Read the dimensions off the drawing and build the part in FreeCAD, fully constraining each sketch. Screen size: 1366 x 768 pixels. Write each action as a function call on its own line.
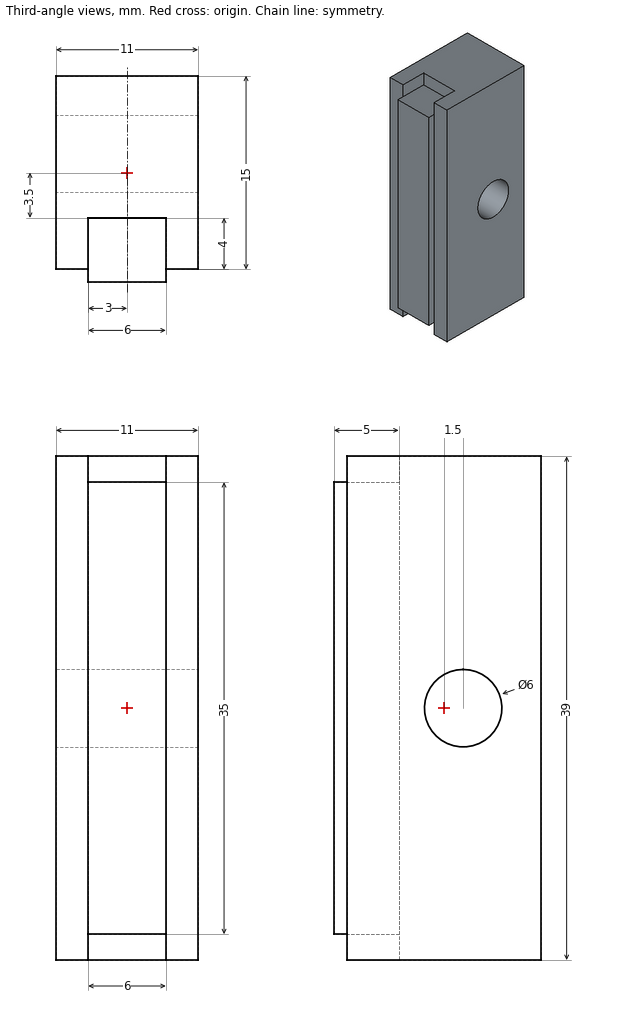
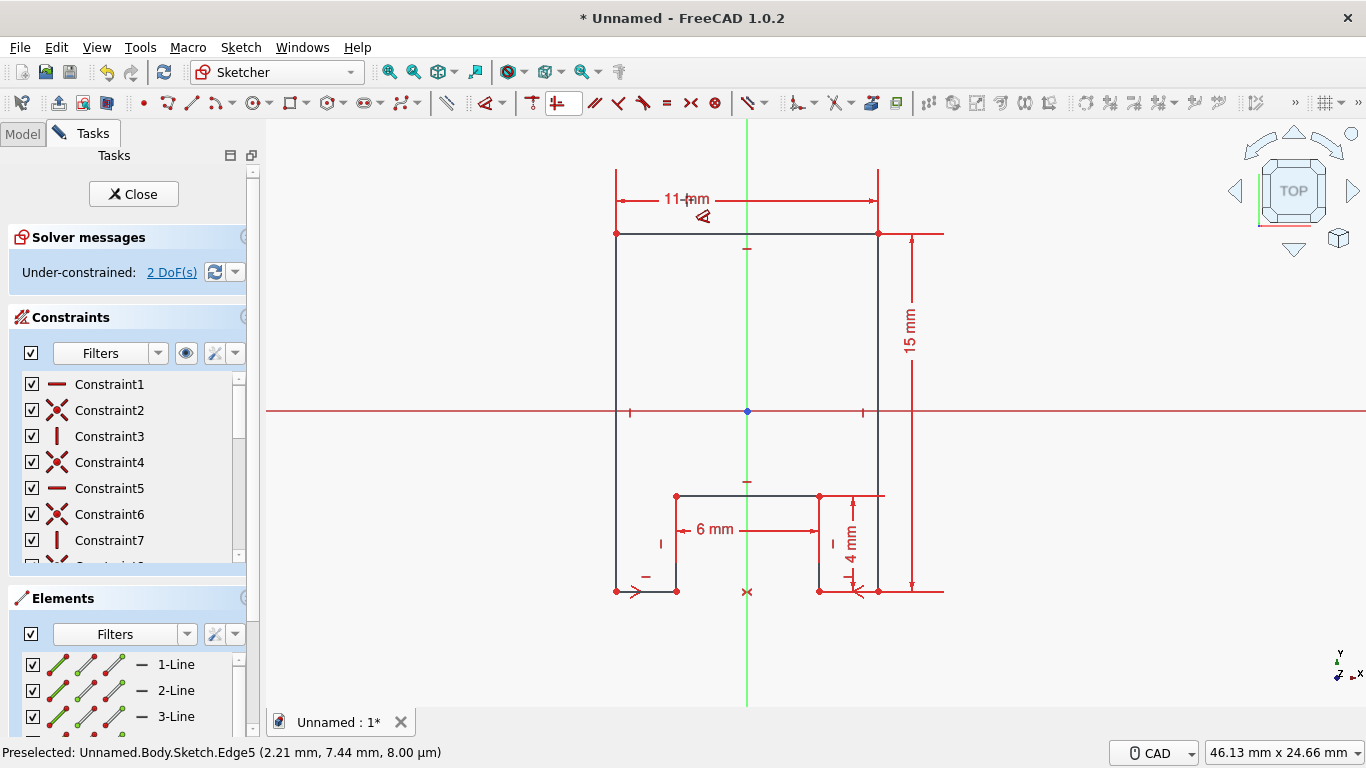
click(676, 496)
click(712, 377)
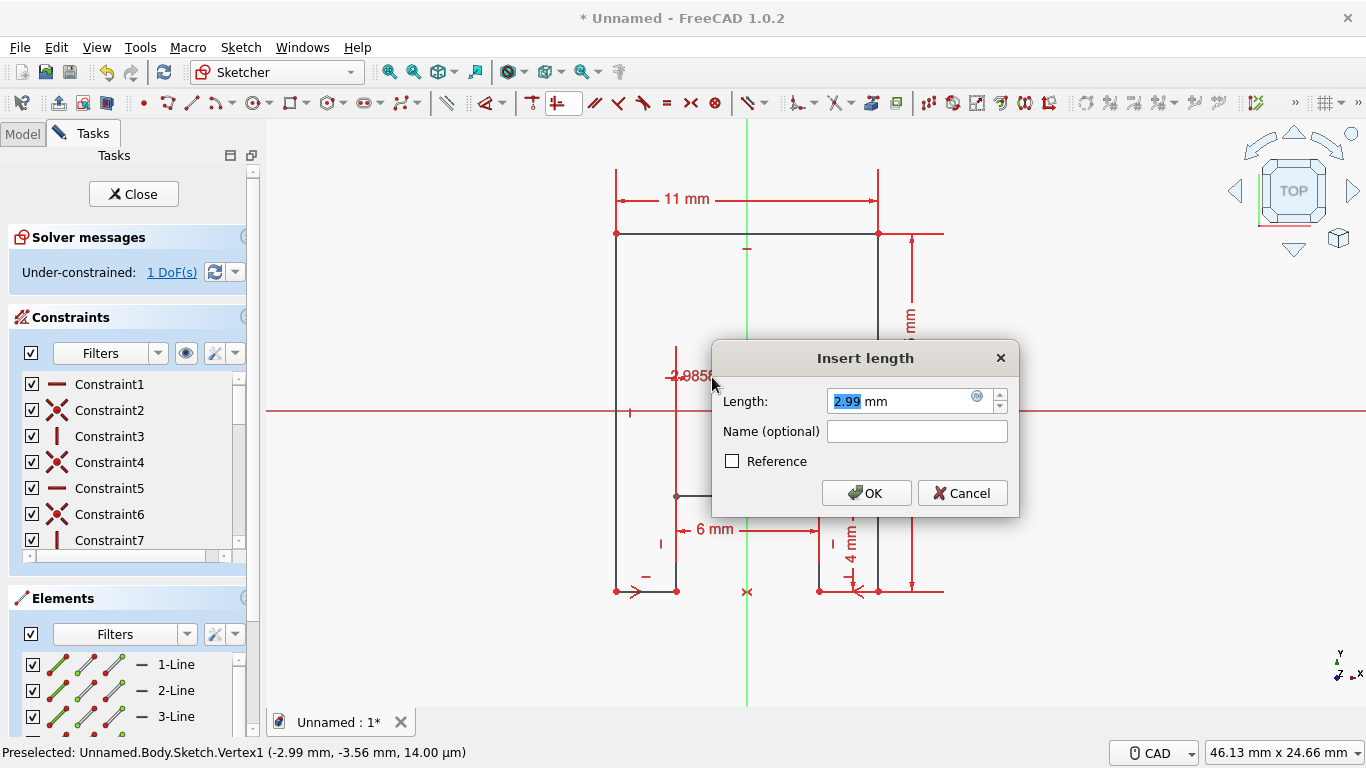
text(3)
key(Return)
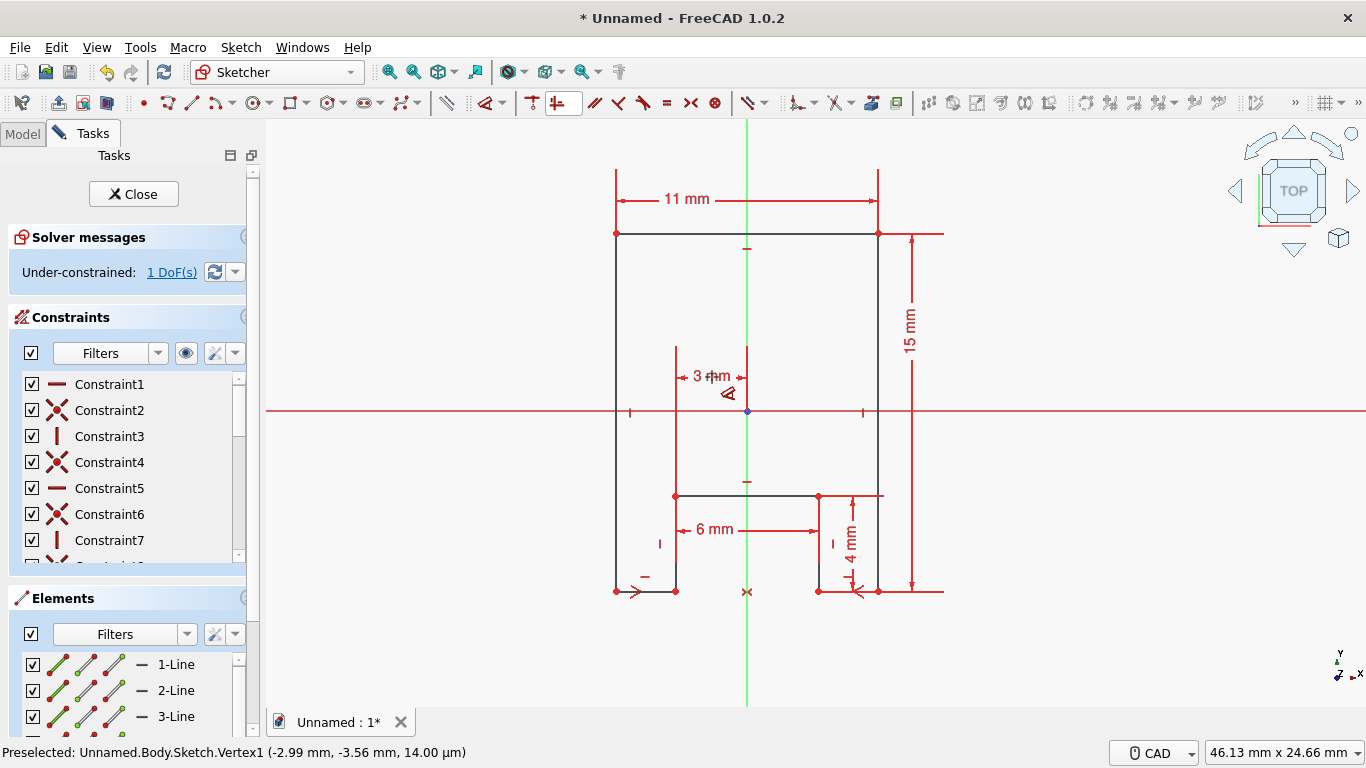
click(676, 496)
click(642, 454)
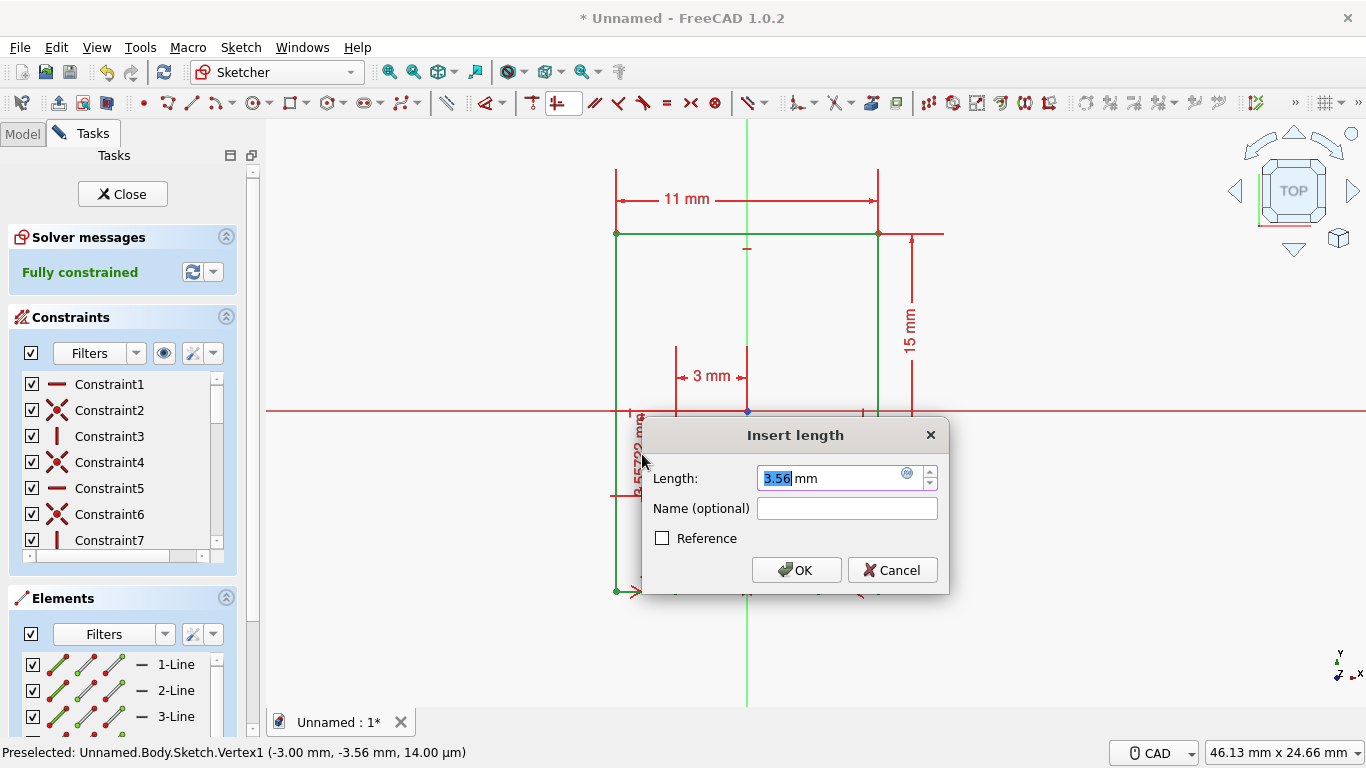
text(3.5)
key(Return)
key(Escape)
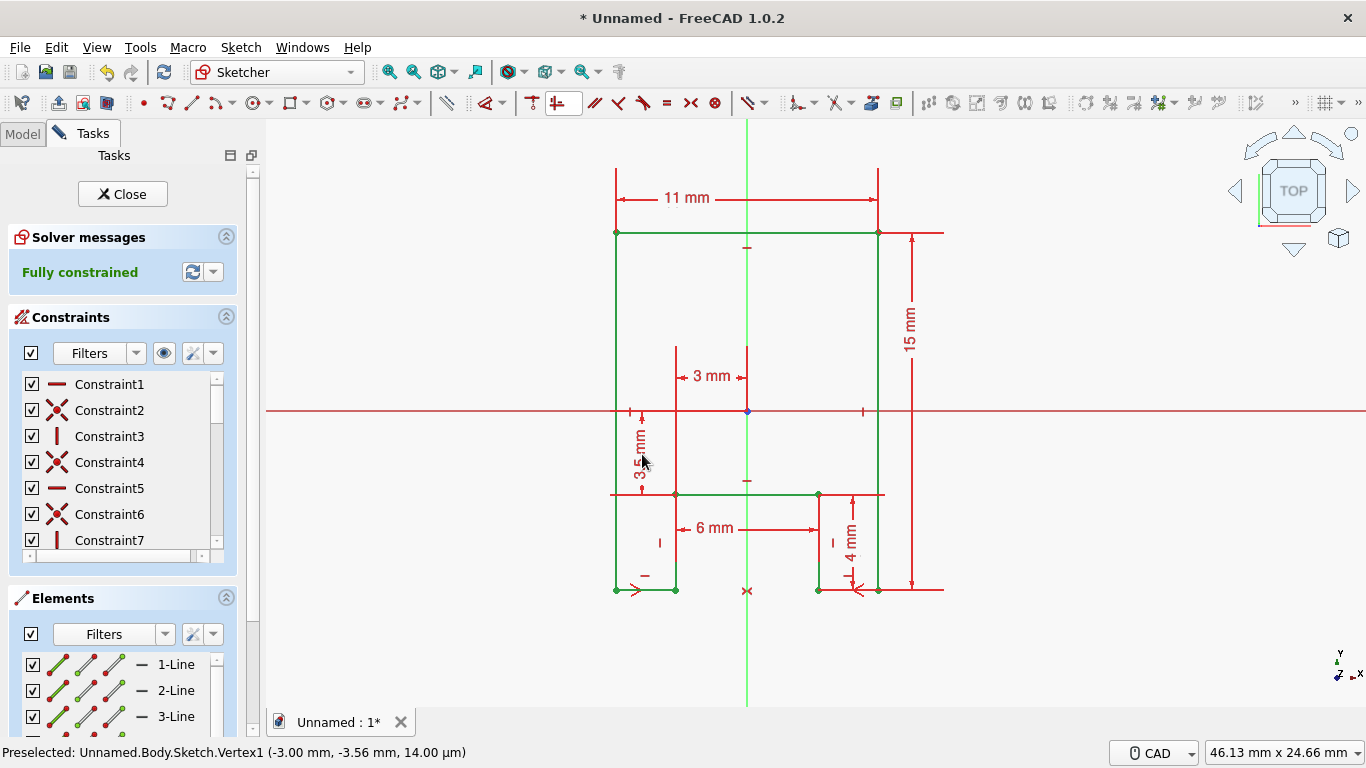
click(123, 194)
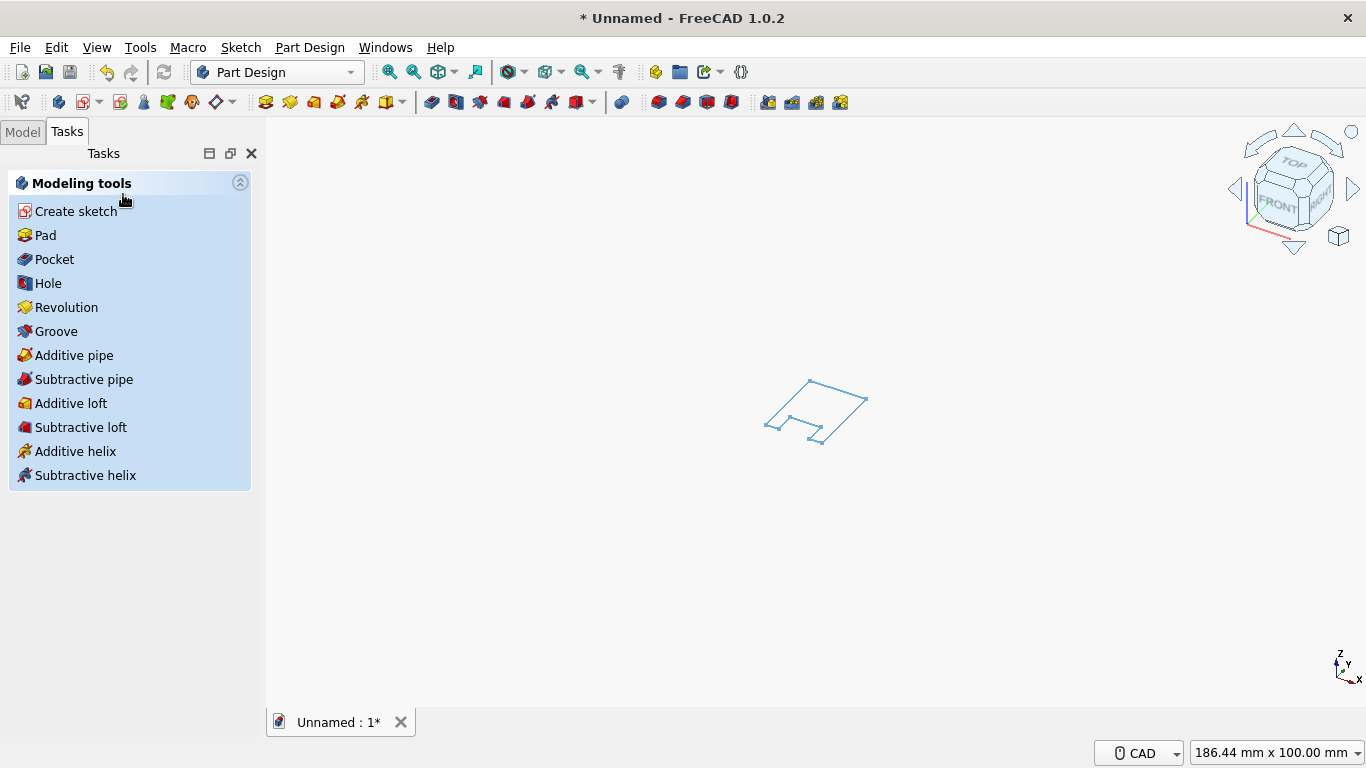
click(266, 102)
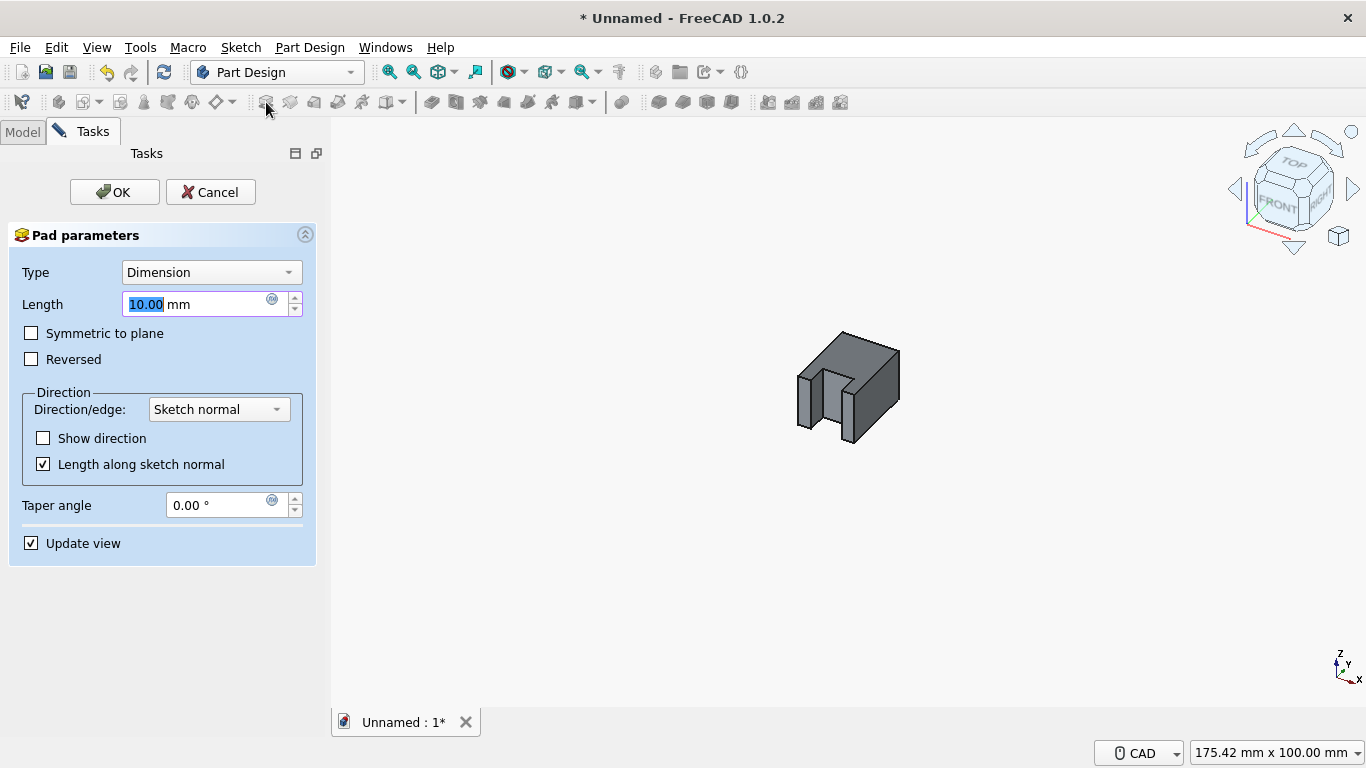
text(39)
key(Tab)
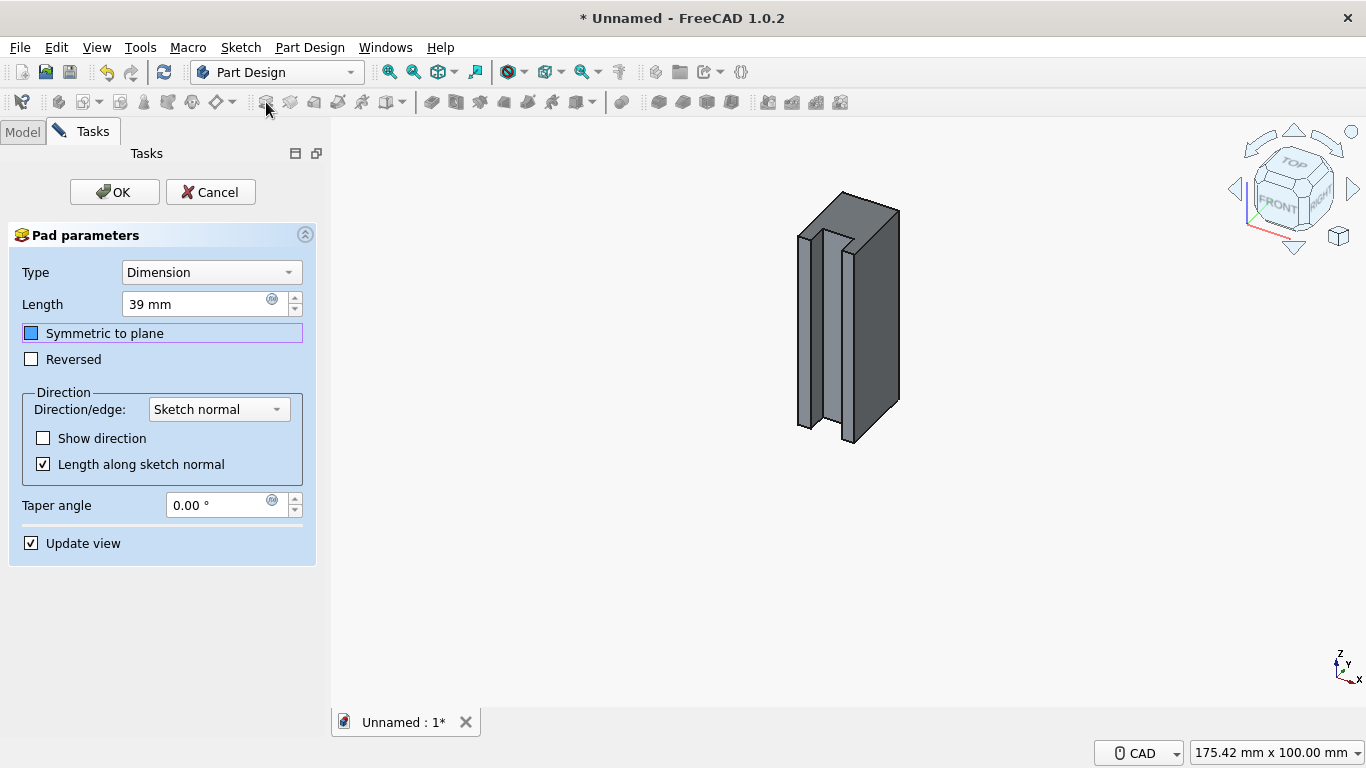
click(30, 333)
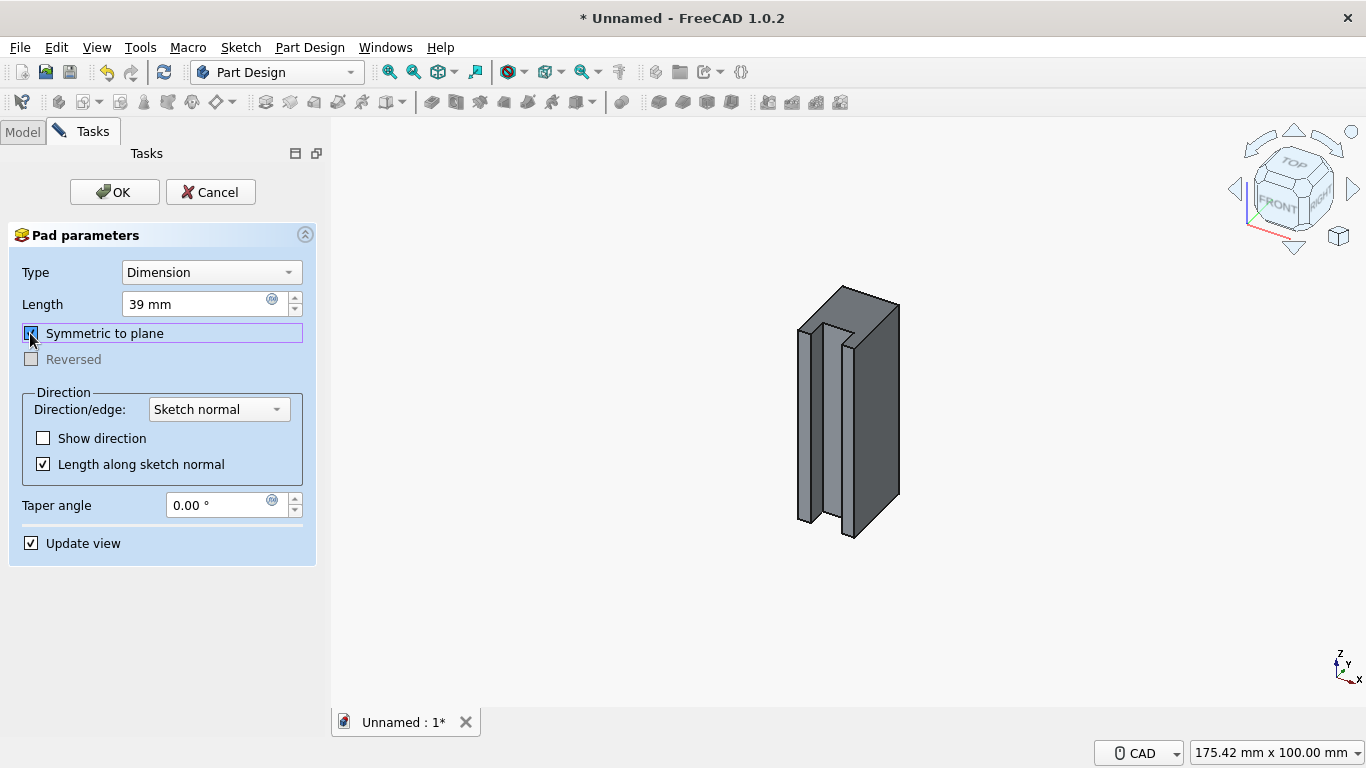
click(115, 192)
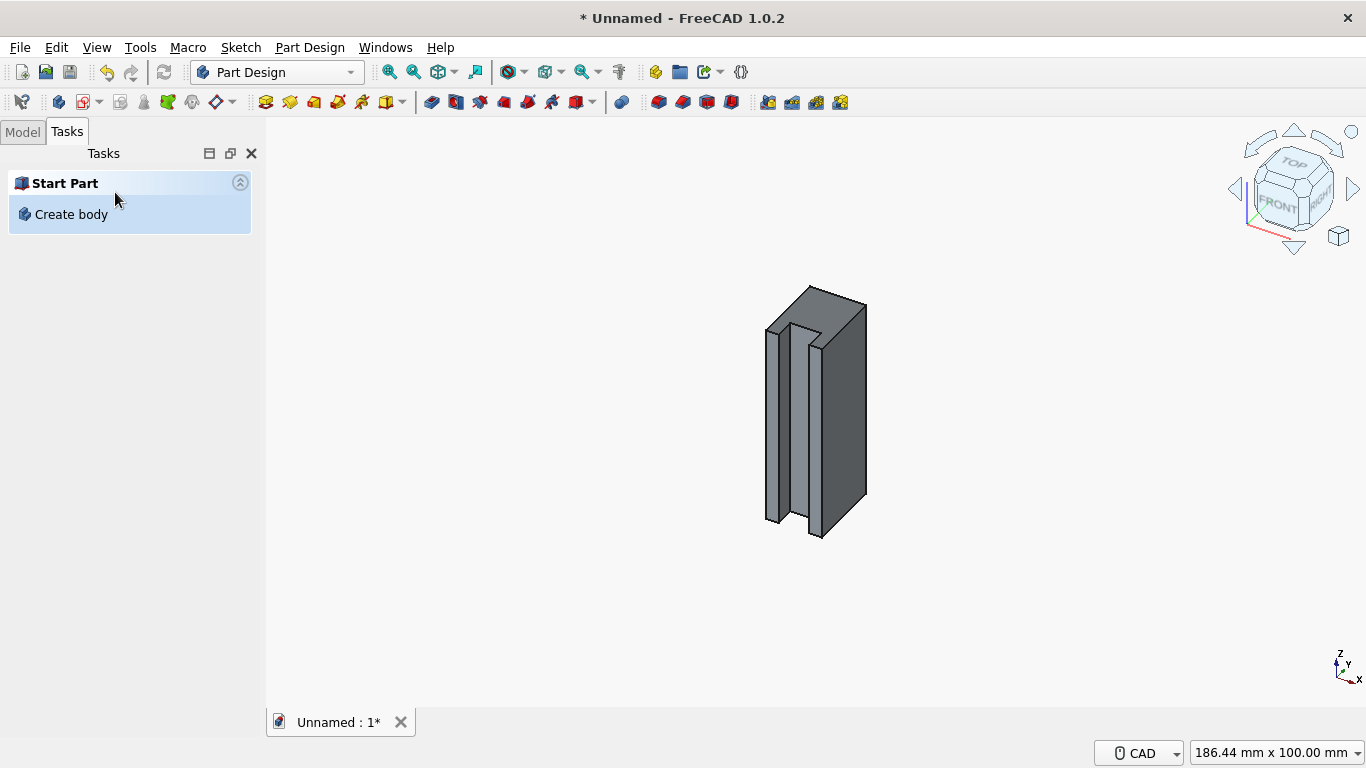
click(390, 72)